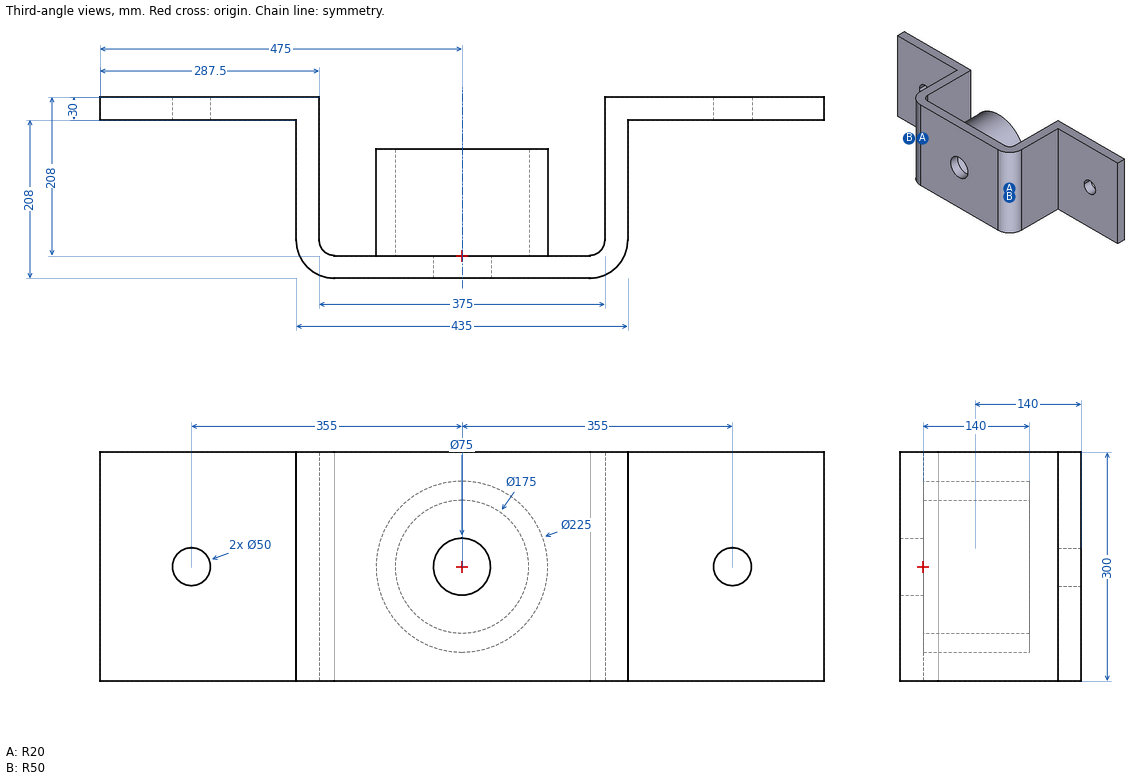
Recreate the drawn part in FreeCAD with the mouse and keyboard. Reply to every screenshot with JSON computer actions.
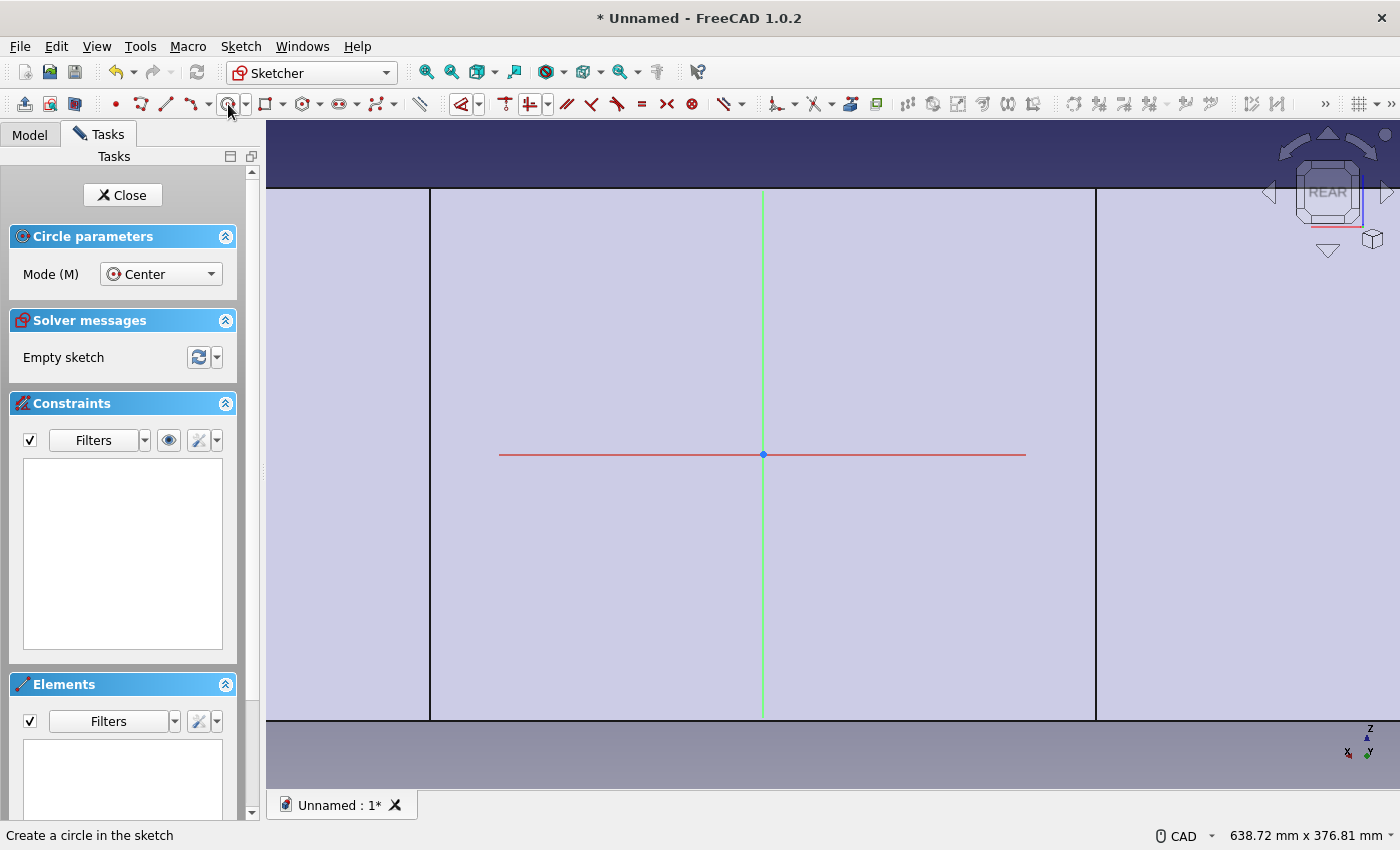
{"action": "left_click", "coordinate": [763, 454]}
{"action": "mouse_move", "coordinate": [905, 313]}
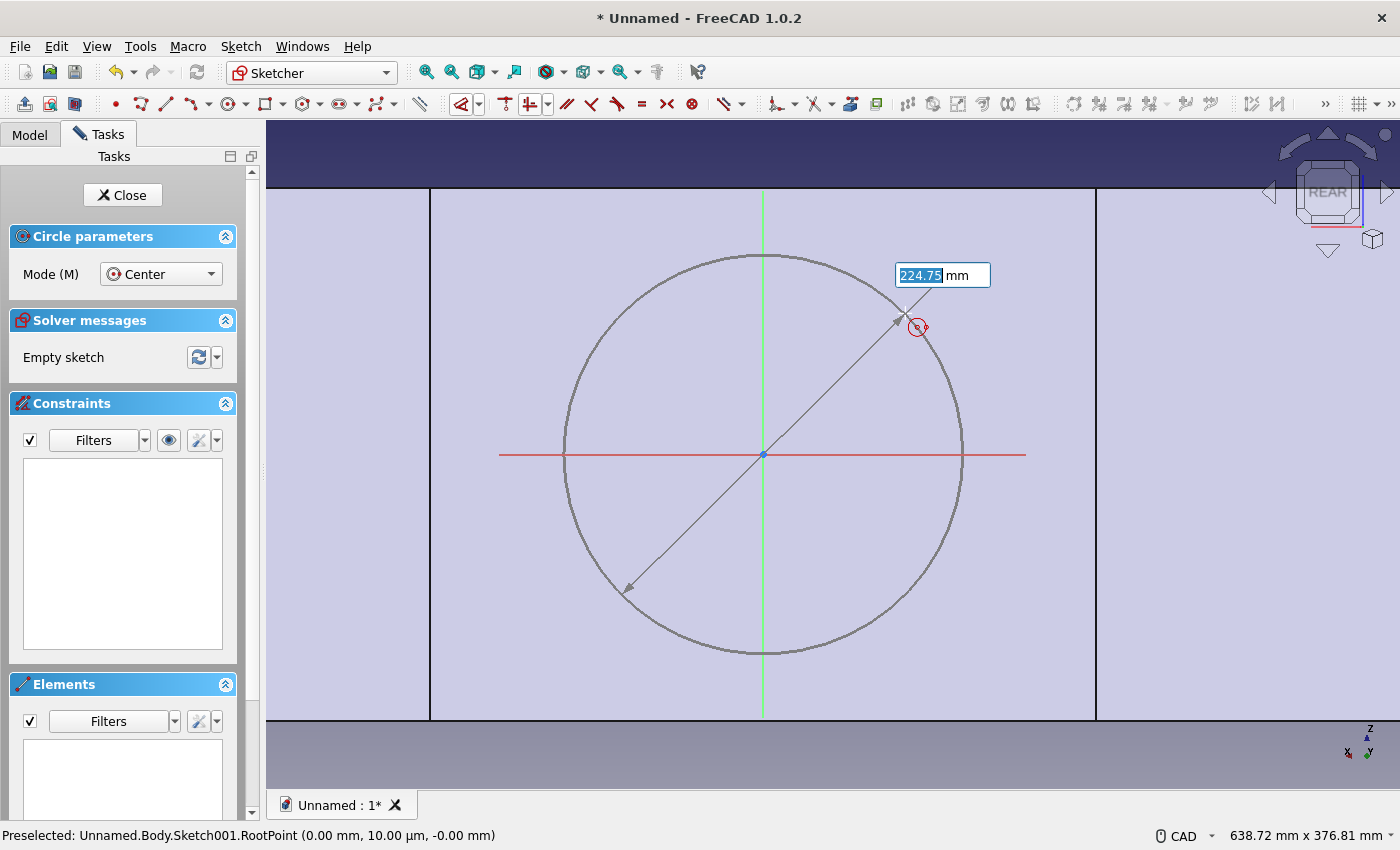
{"action": "type", "text": "225"}
{"action": "key", "text": "Return"}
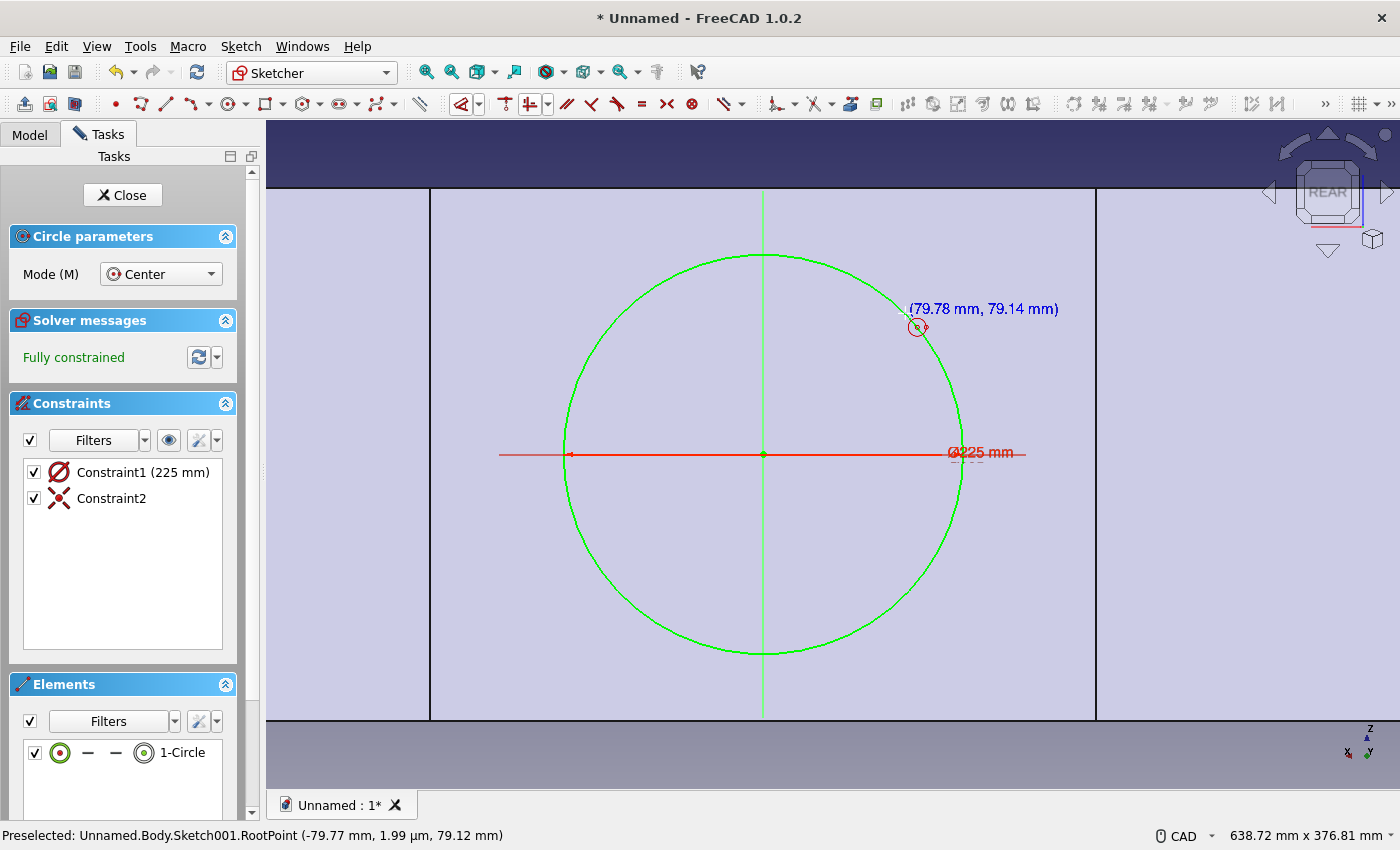
{"action": "left_click", "coordinate": [763, 454]}
{"action": "mouse_move", "coordinate": [873, 345]}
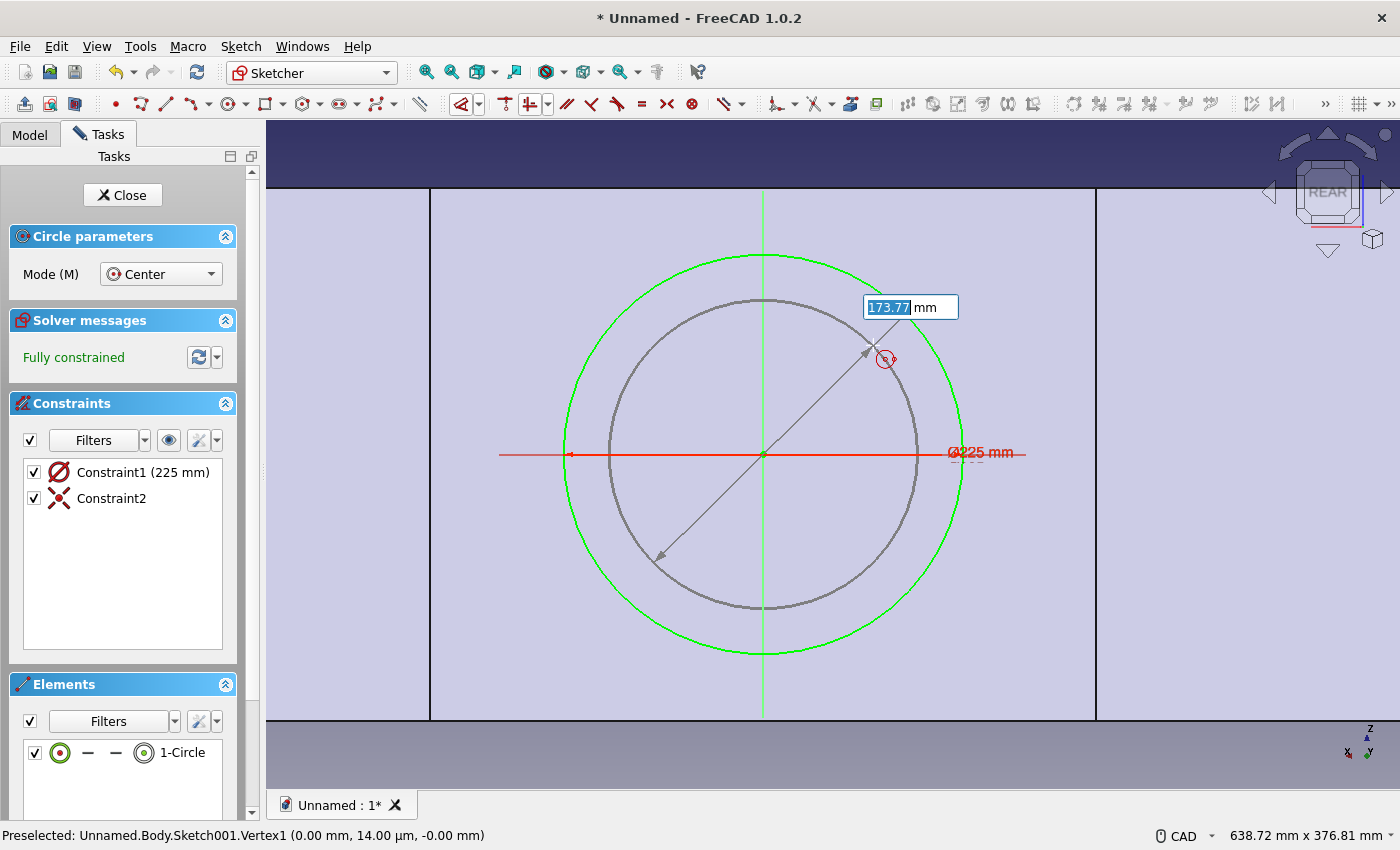
{"action": "type", "text": "175"}
{"action": "key", "text": "Return"}
{"action": "key", "text": "Escape"}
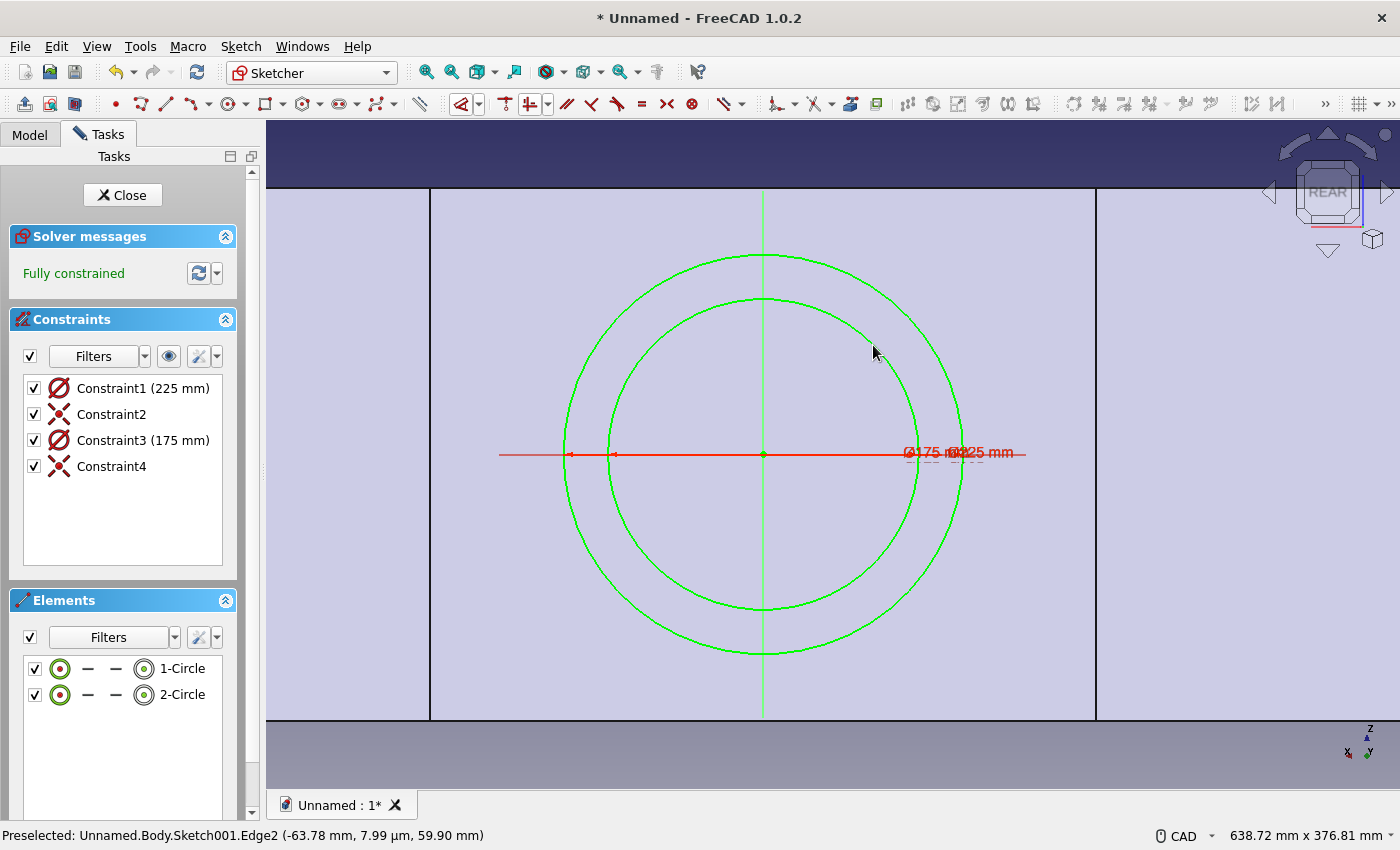
{"action": "left_click", "coordinate": [123, 195]}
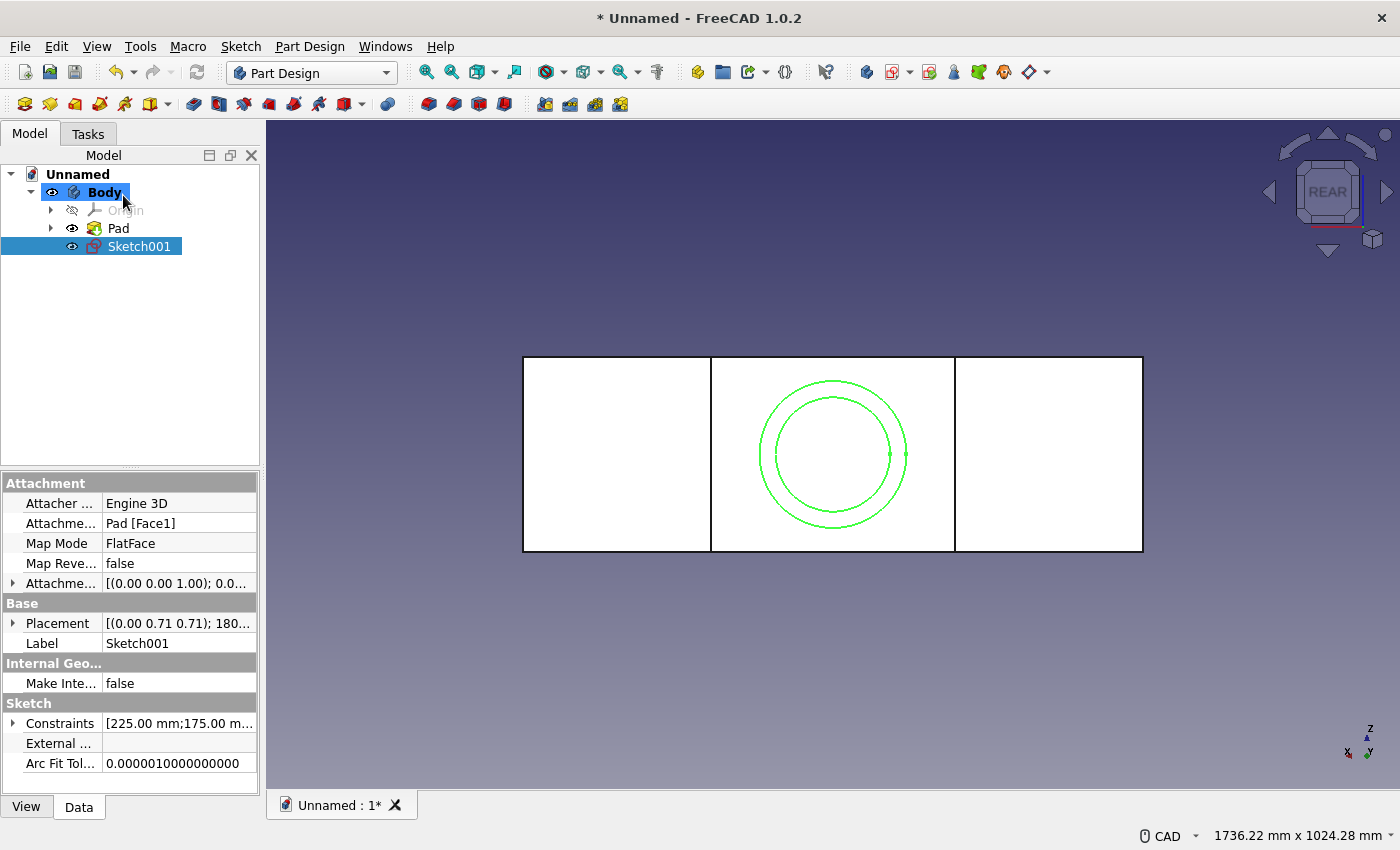
{"action": "left_click", "coordinate": [25, 104]}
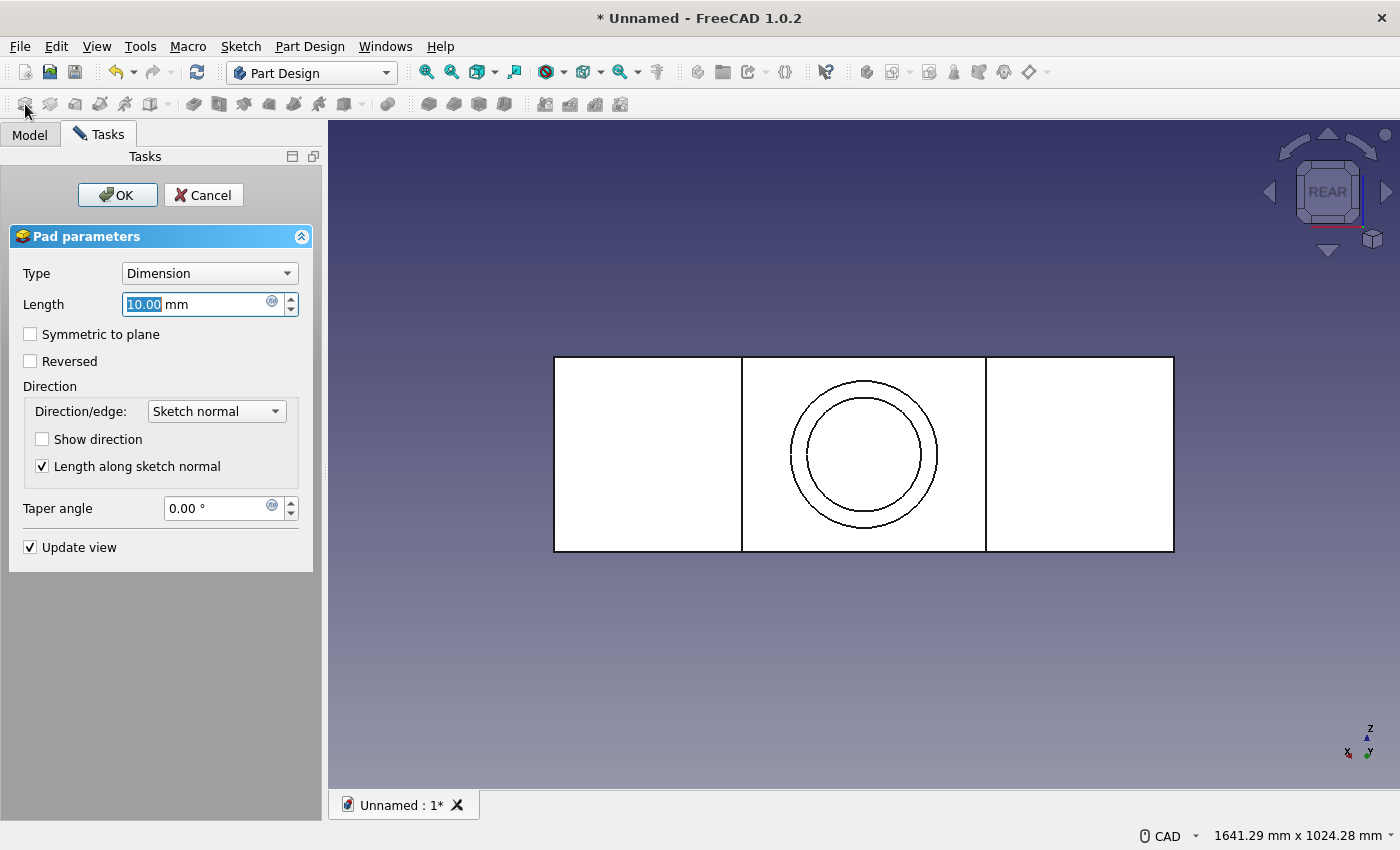
{"action": "type", "text": "140"}
{"action": "key", "text": "Tab"}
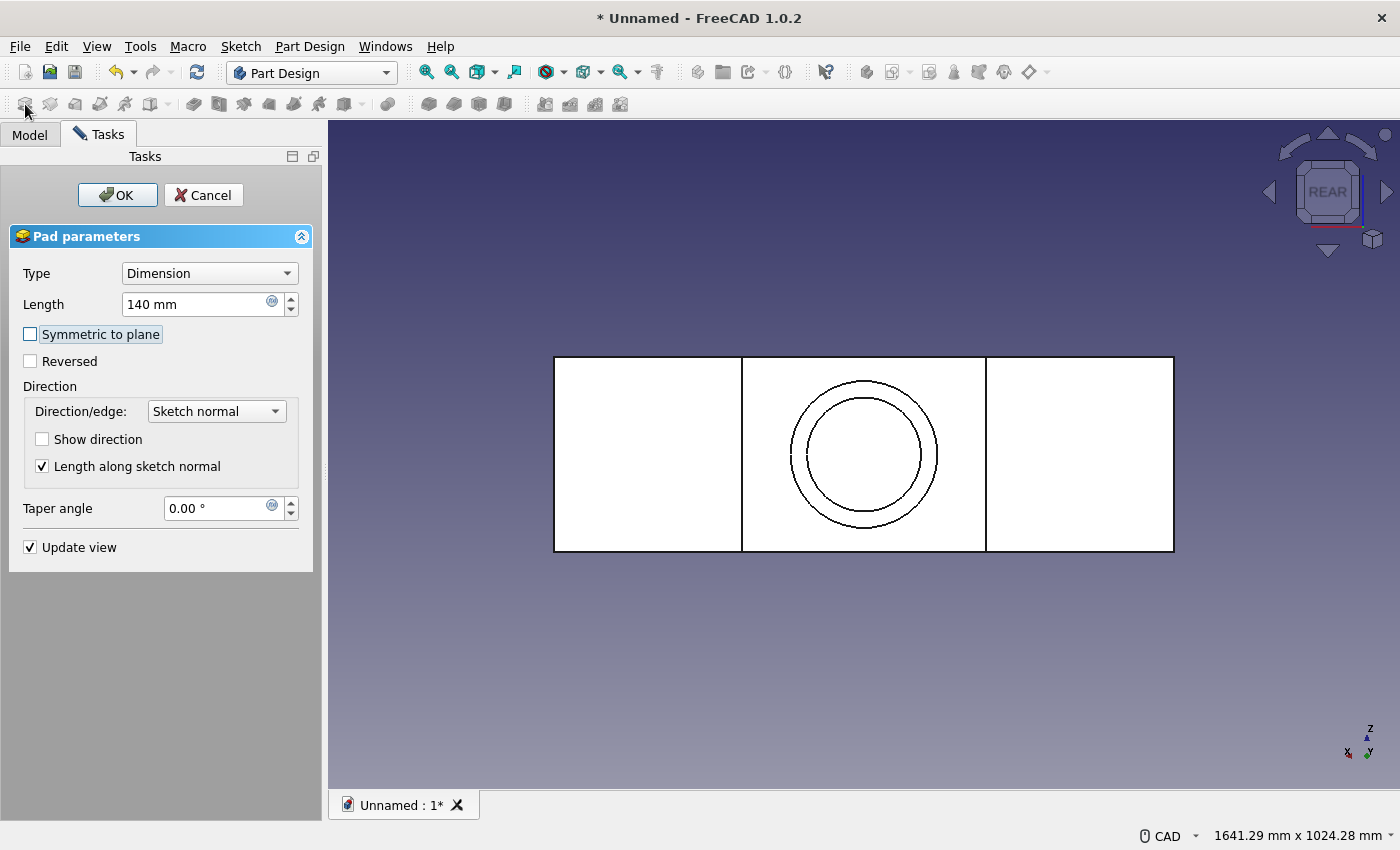
{"action": "left_click", "coordinate": [118, 195]}